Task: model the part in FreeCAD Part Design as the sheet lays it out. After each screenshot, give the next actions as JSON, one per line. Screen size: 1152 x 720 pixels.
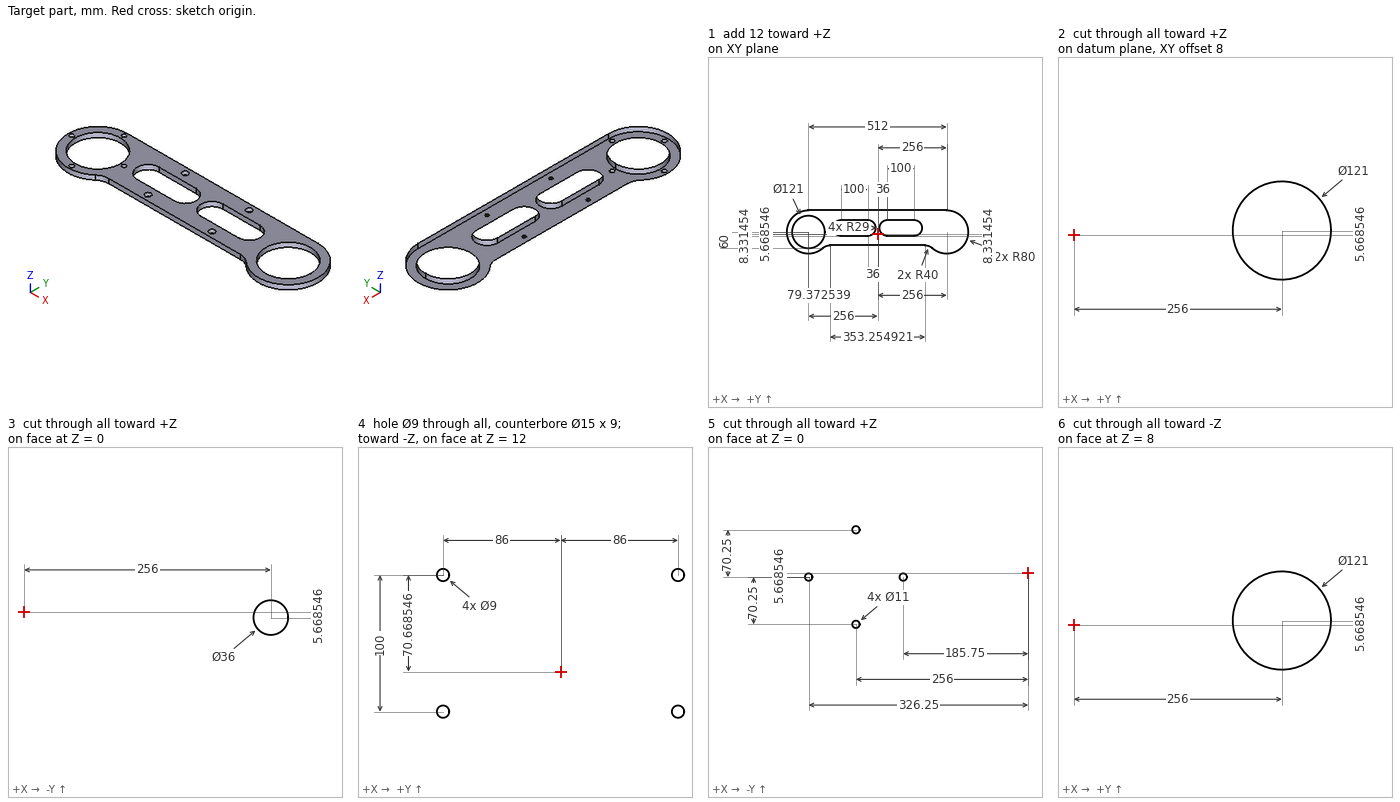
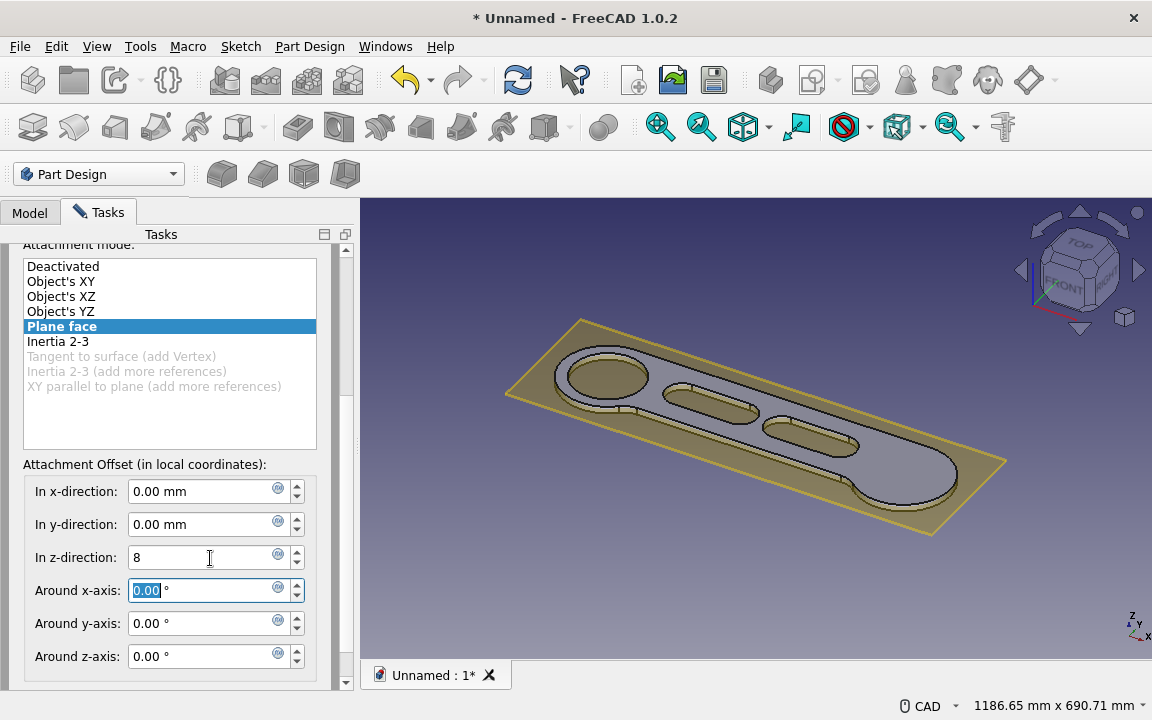
{"action": "scroll", "coordinate": [346, 467], "scroll_direction": "up", "scroll_amount": 5}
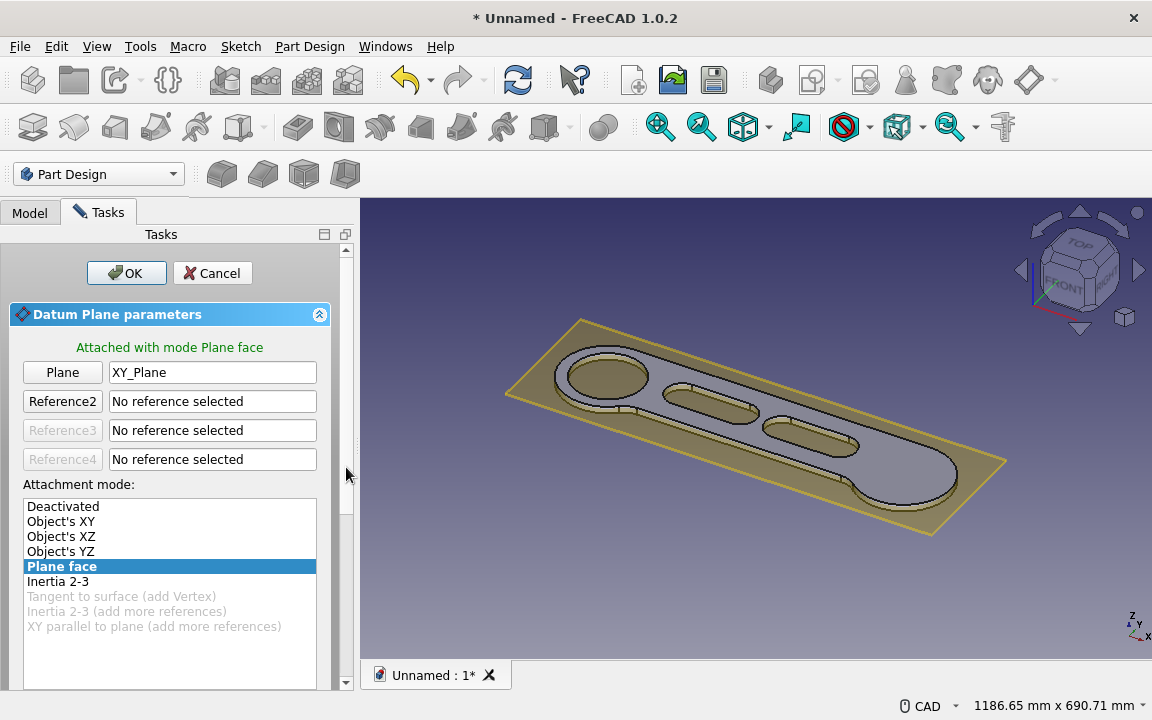
{"action": "left_click", "coordinate": [127, 273]}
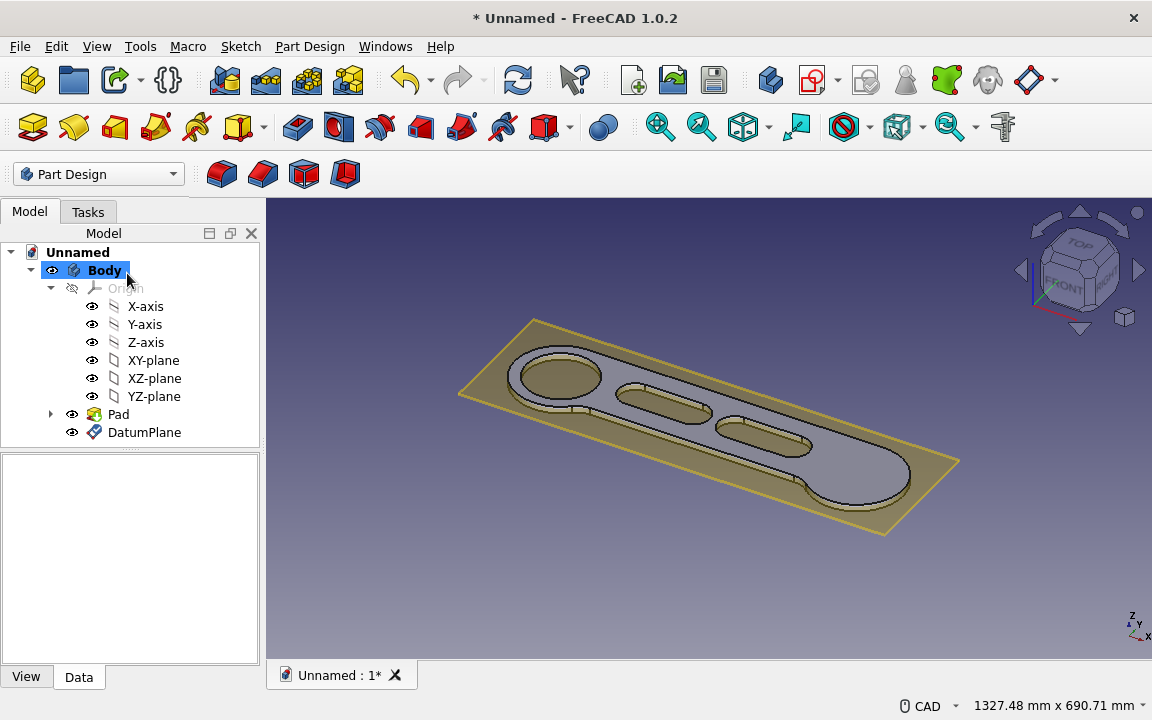
{"action": "left_click", "coordinate": [117, 432]}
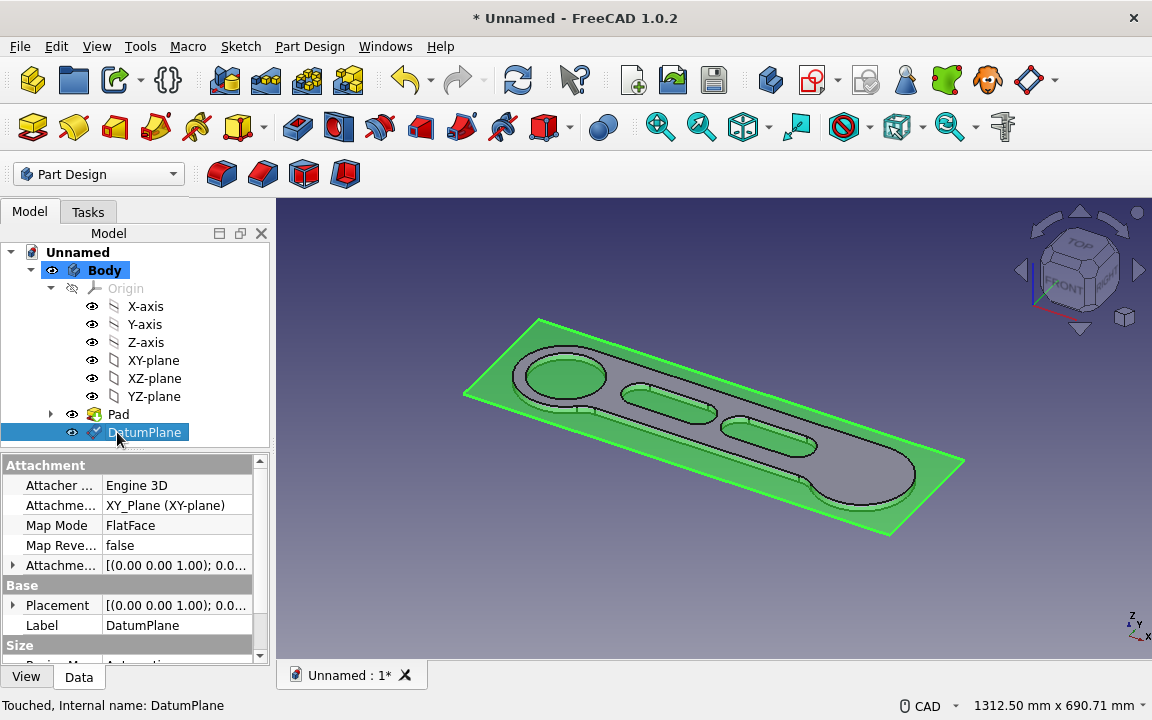
{"action": "left_click", "coordinate": [812, 80]}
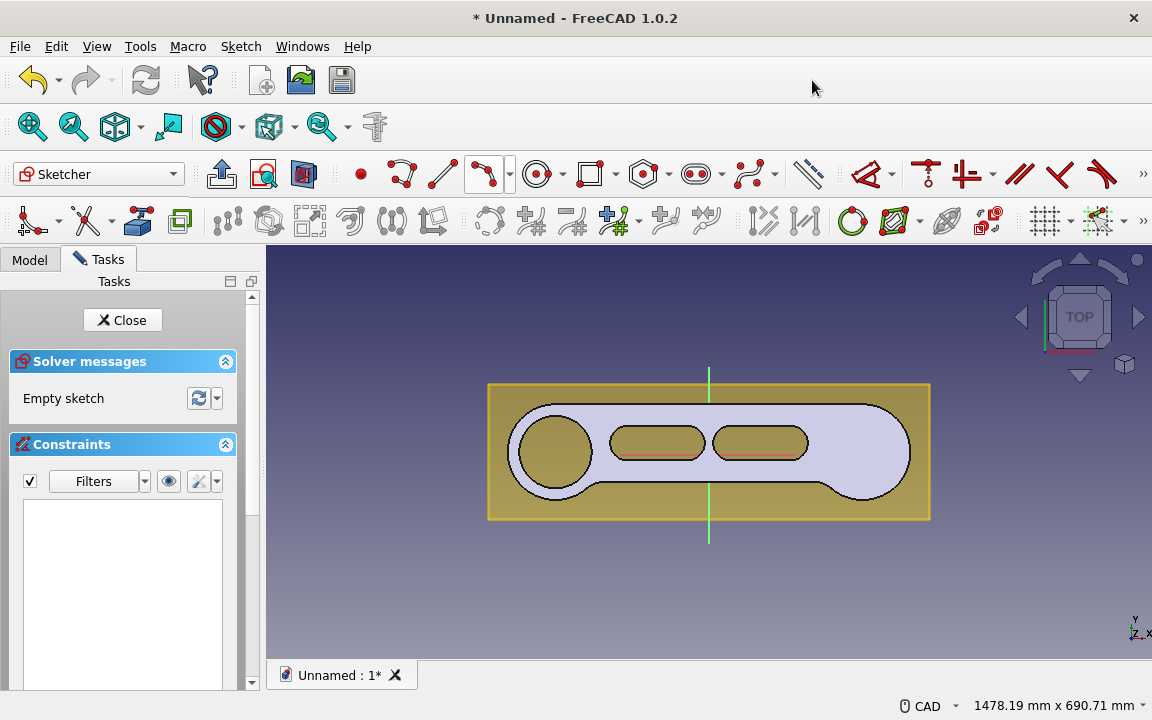
{"action": "left_click", "coordinate": [304, 174]}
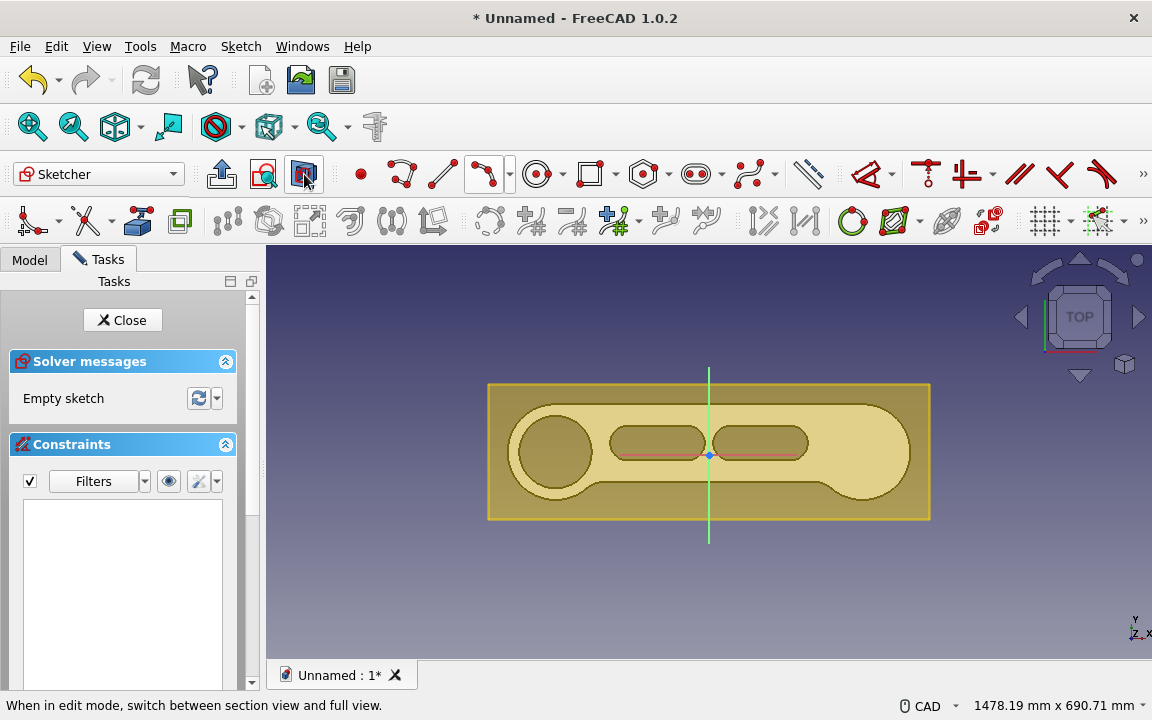
{"action": "scroll", "coordinate": [958, 452], "scroll_direction": "up", "scroll_amount": 6}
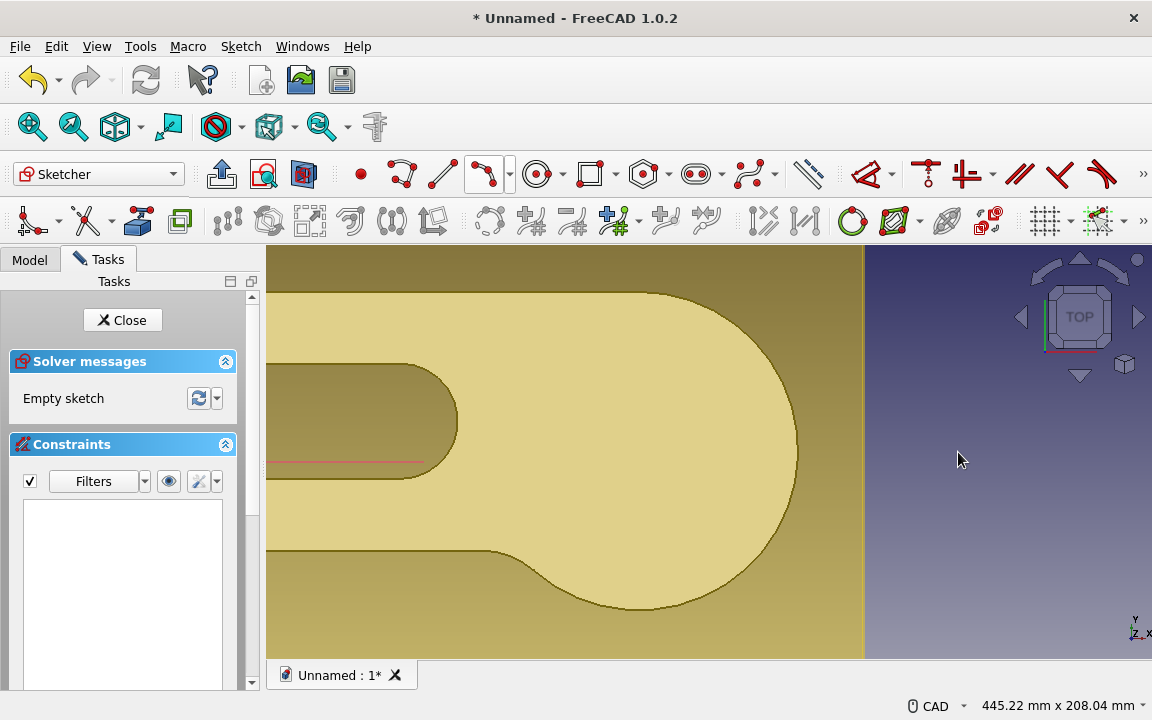
{"action": "left_click", "coordinate": [536, 174]}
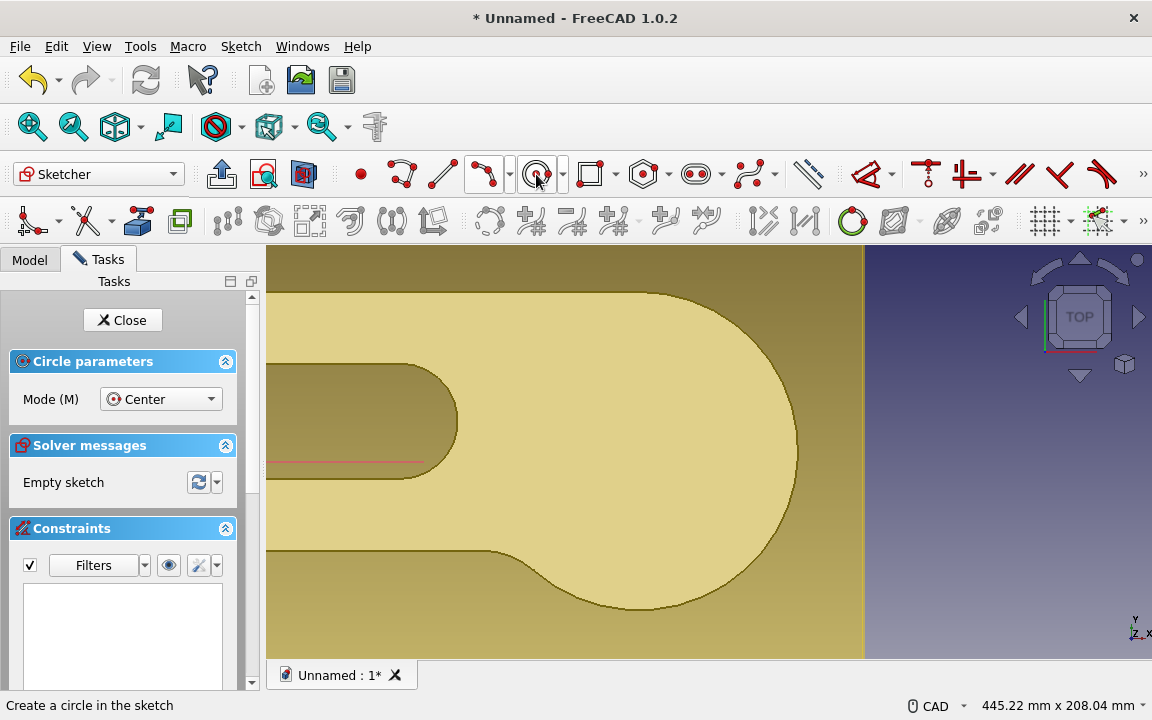
{"action": "scroll", "coordinate": [639, 451], "scroll_direction": "up", "scroll_amount": 2}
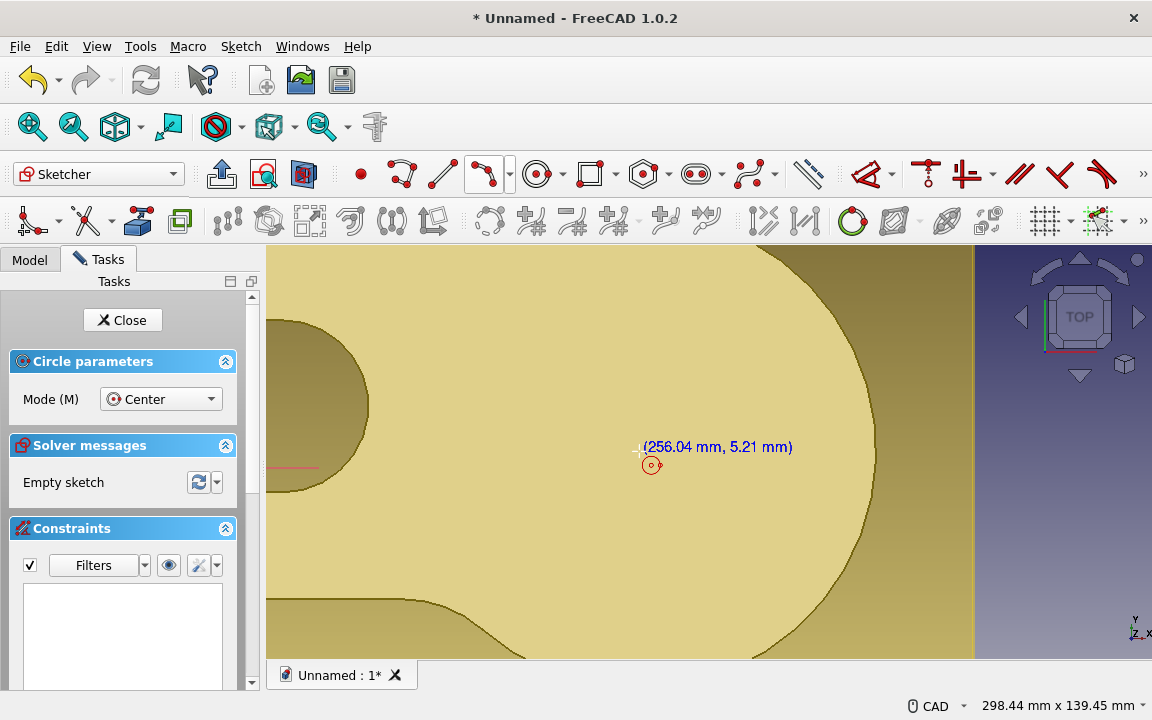
{"action": "left_click", "coordinate": [639, 451]}
{"action": "mouse_move", "coordinate": [766, 324]}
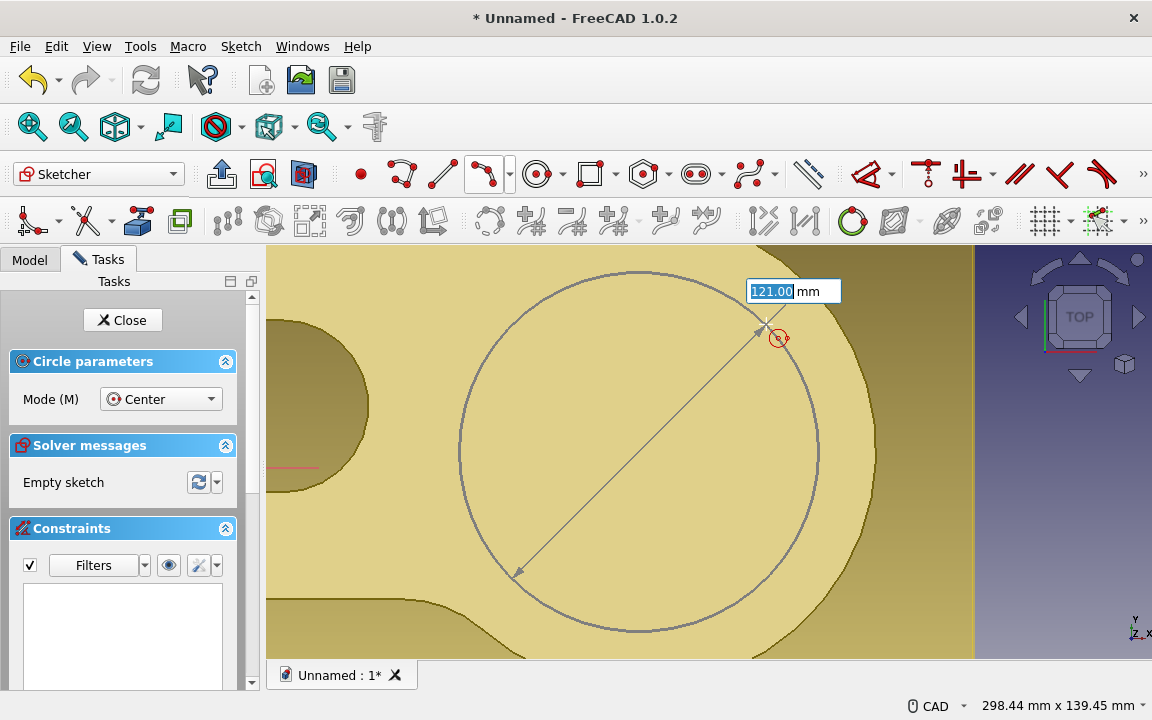
{"action": "type", "text": "121"}
{"action": "key", "text": "Return"}
{"action": "key", "text": "Escape"}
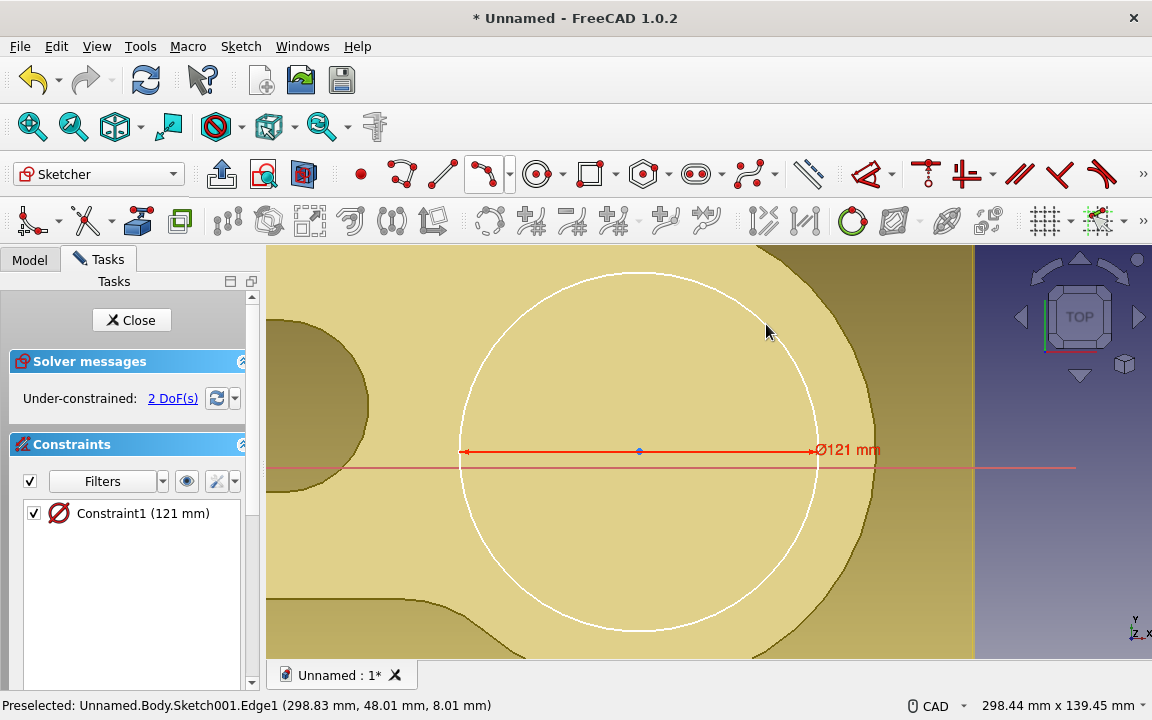
{"action": "left_click", "coordinate": [866, 174]}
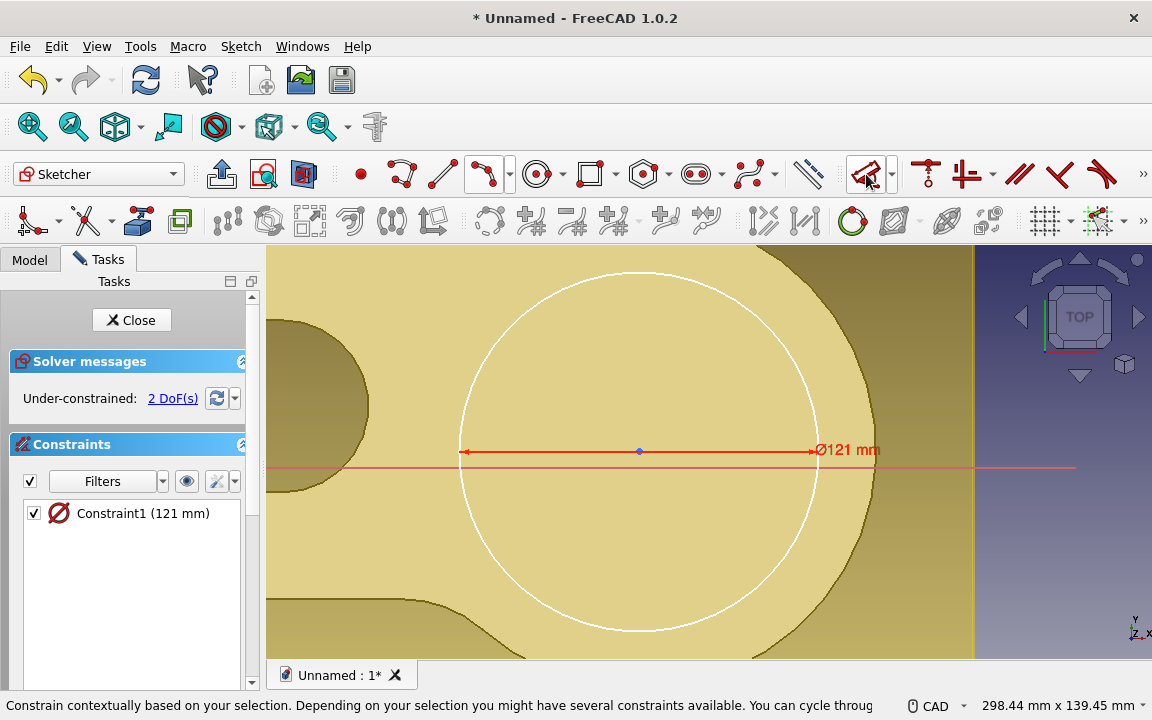
{"action": "left_click", "coordinate": [639, 452]}
{"action": "left_click", "coordinate": [387, 502]}